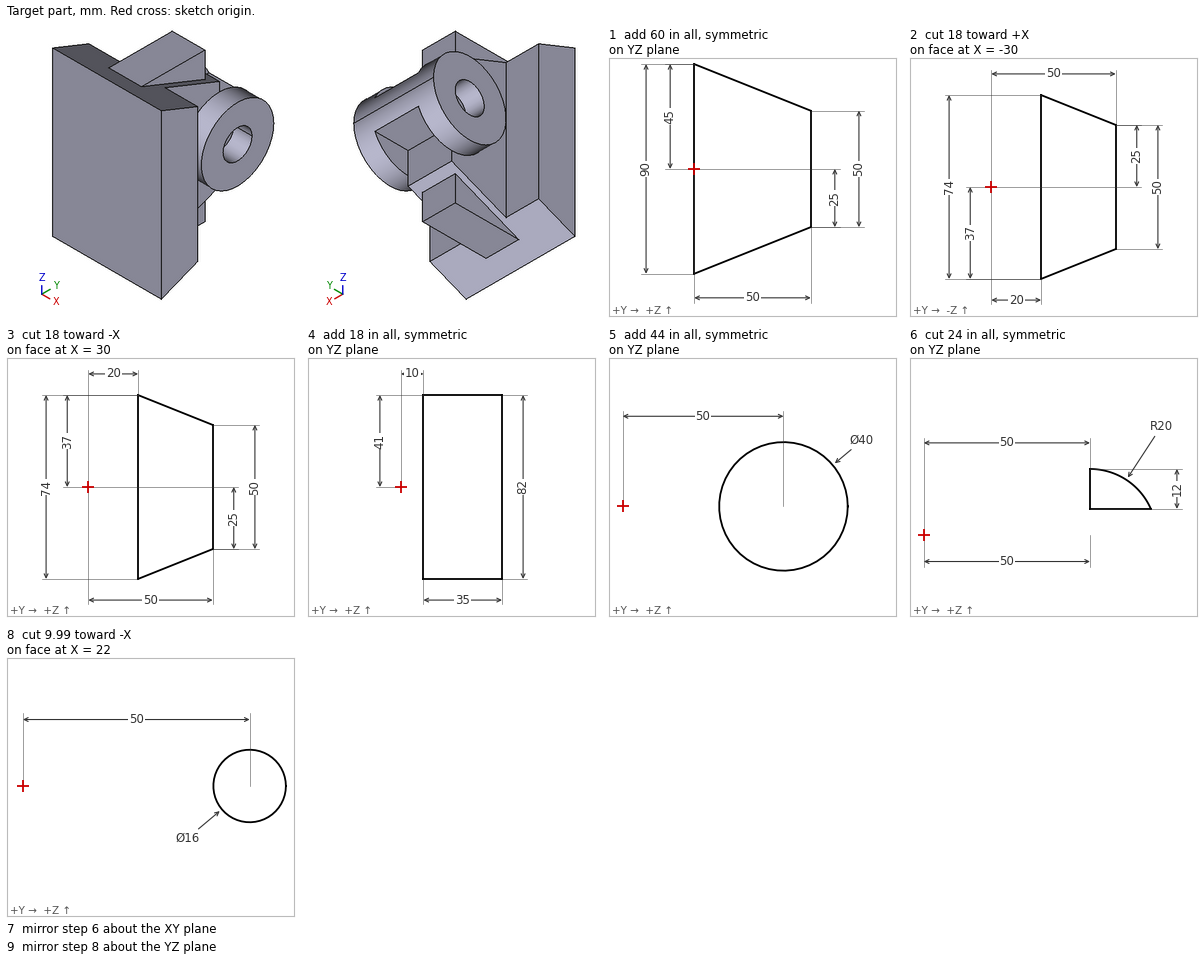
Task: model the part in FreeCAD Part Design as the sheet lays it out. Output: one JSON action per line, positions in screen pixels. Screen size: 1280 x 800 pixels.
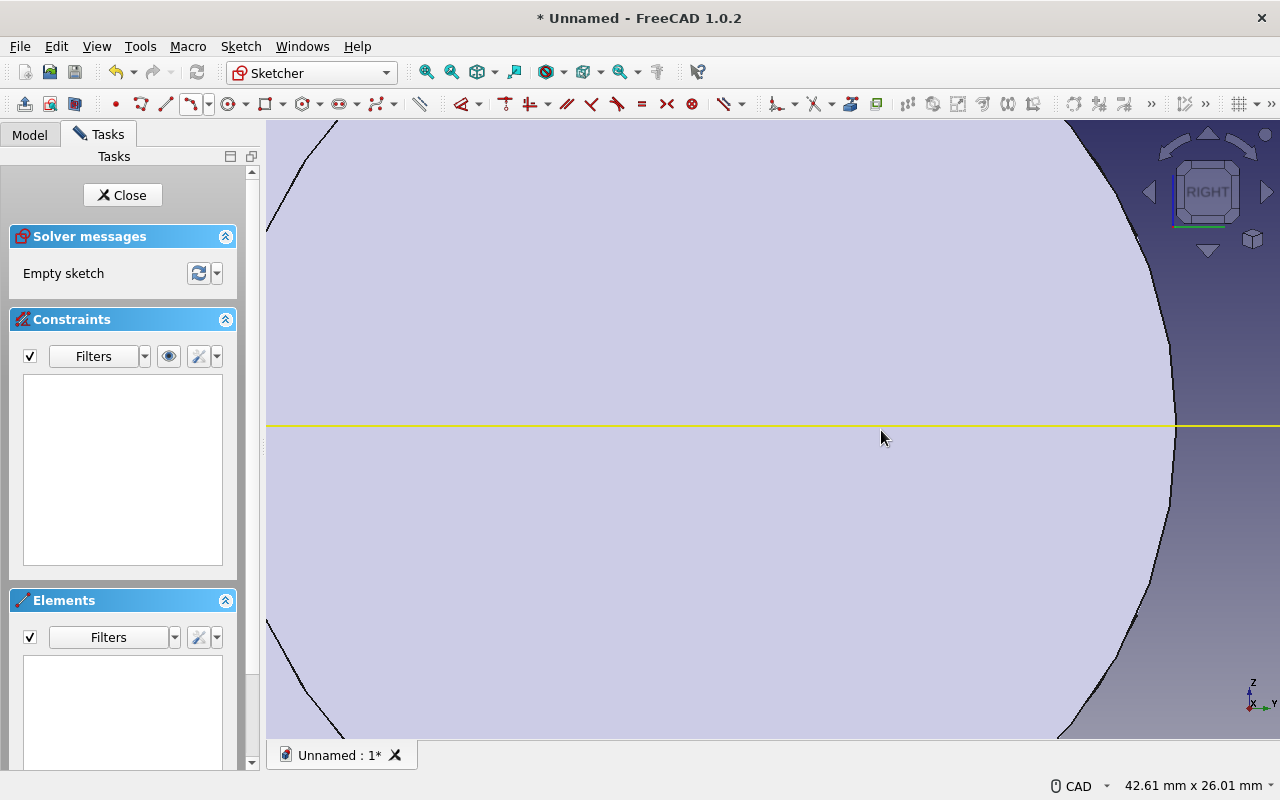
{"action": "left_click", "coordinate": [228, 104]}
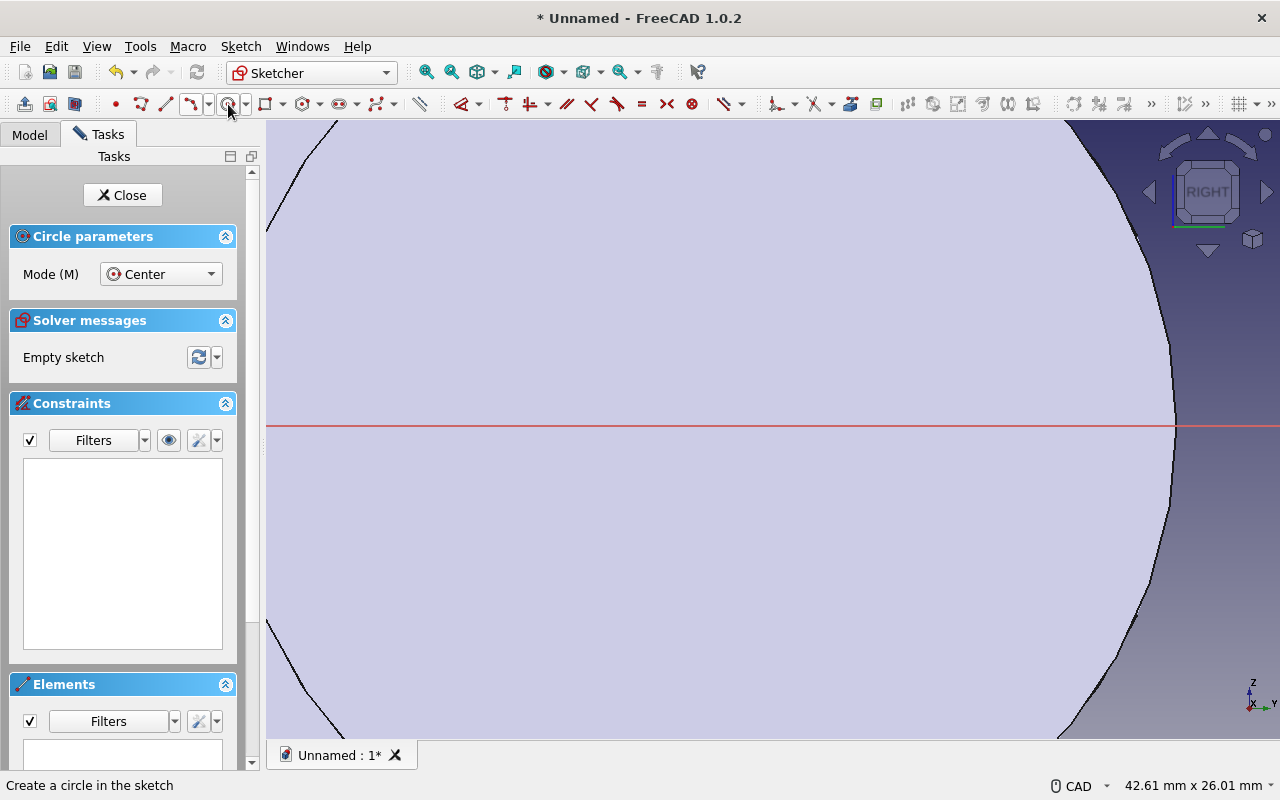
{"action": "left_click", "coordinate": [701, 426]}
{"action": "mouse_move", "coordinate": [835, 291]}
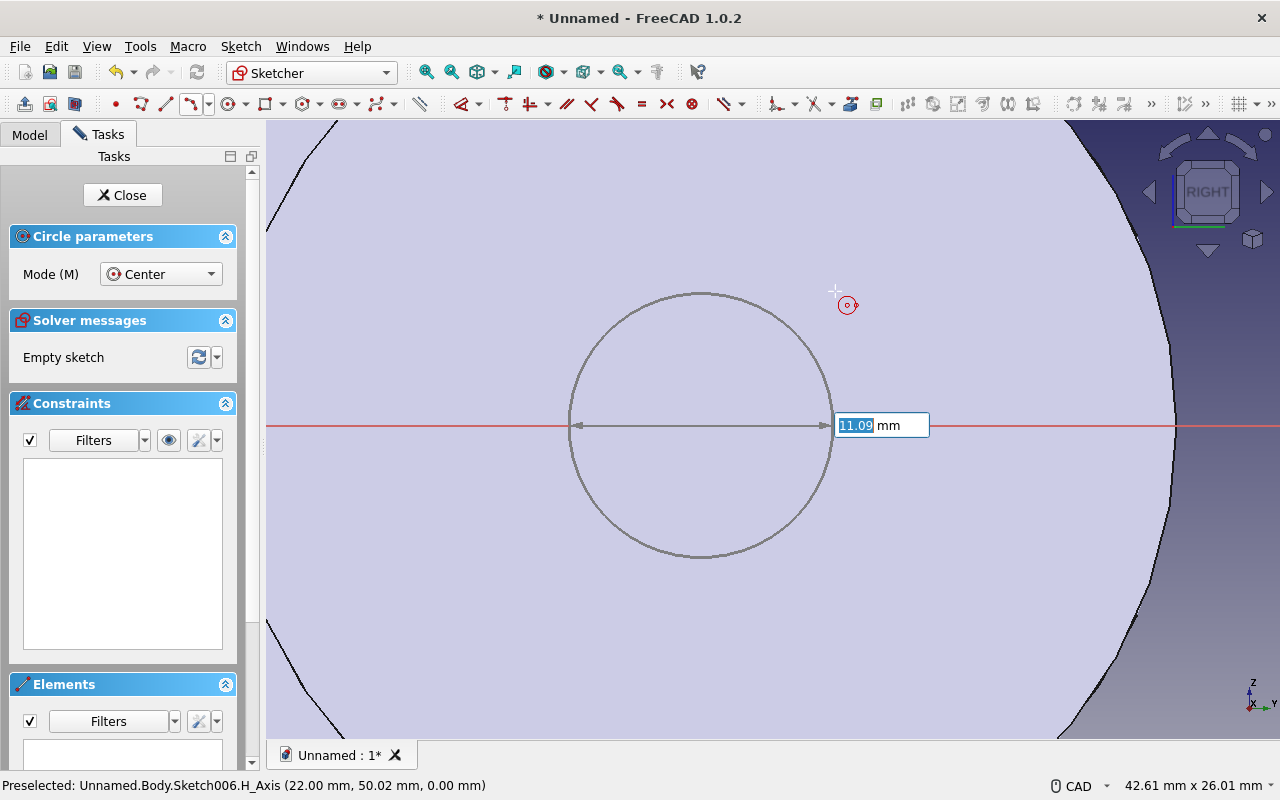
{"action": "type", "text": "16"}
{"action": "key", "text": "Return"}
{"action": "key", "text": "Escape"}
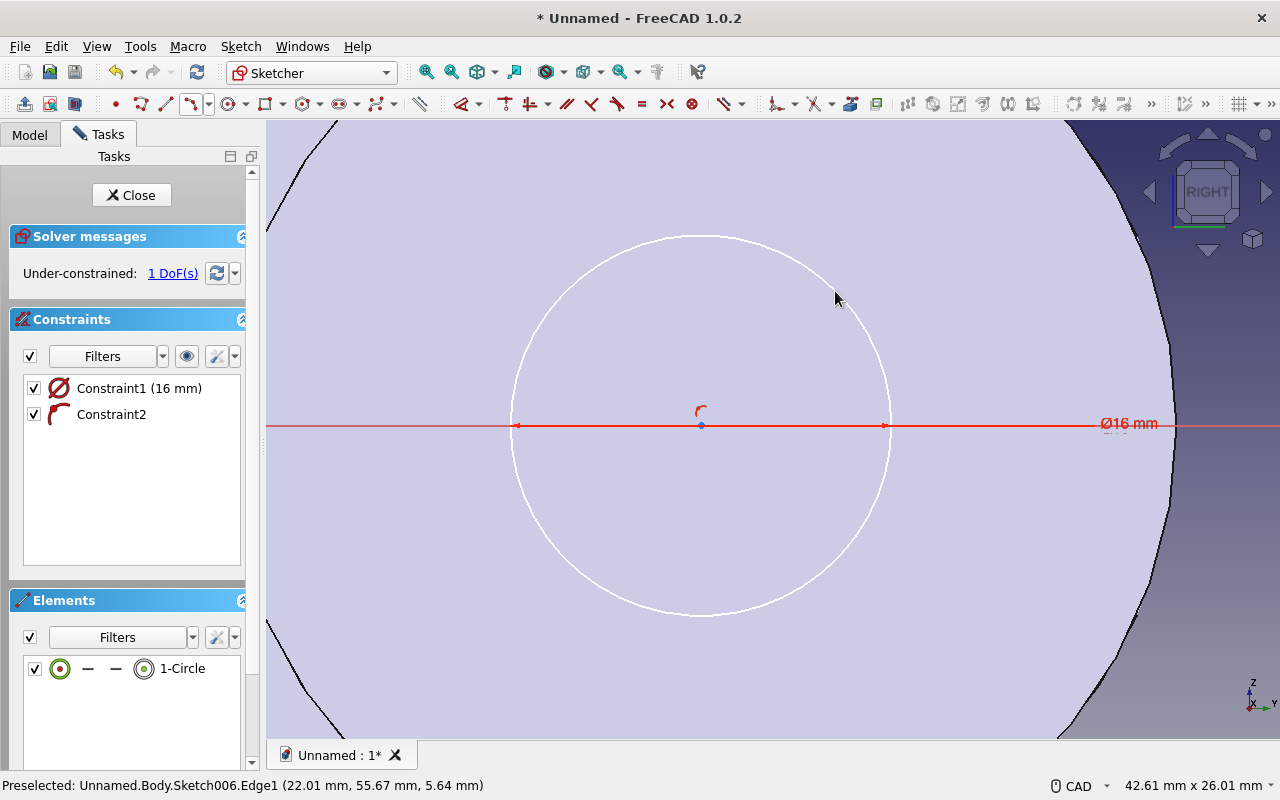
{"action": "left_click", "coordinate": [460, 104]}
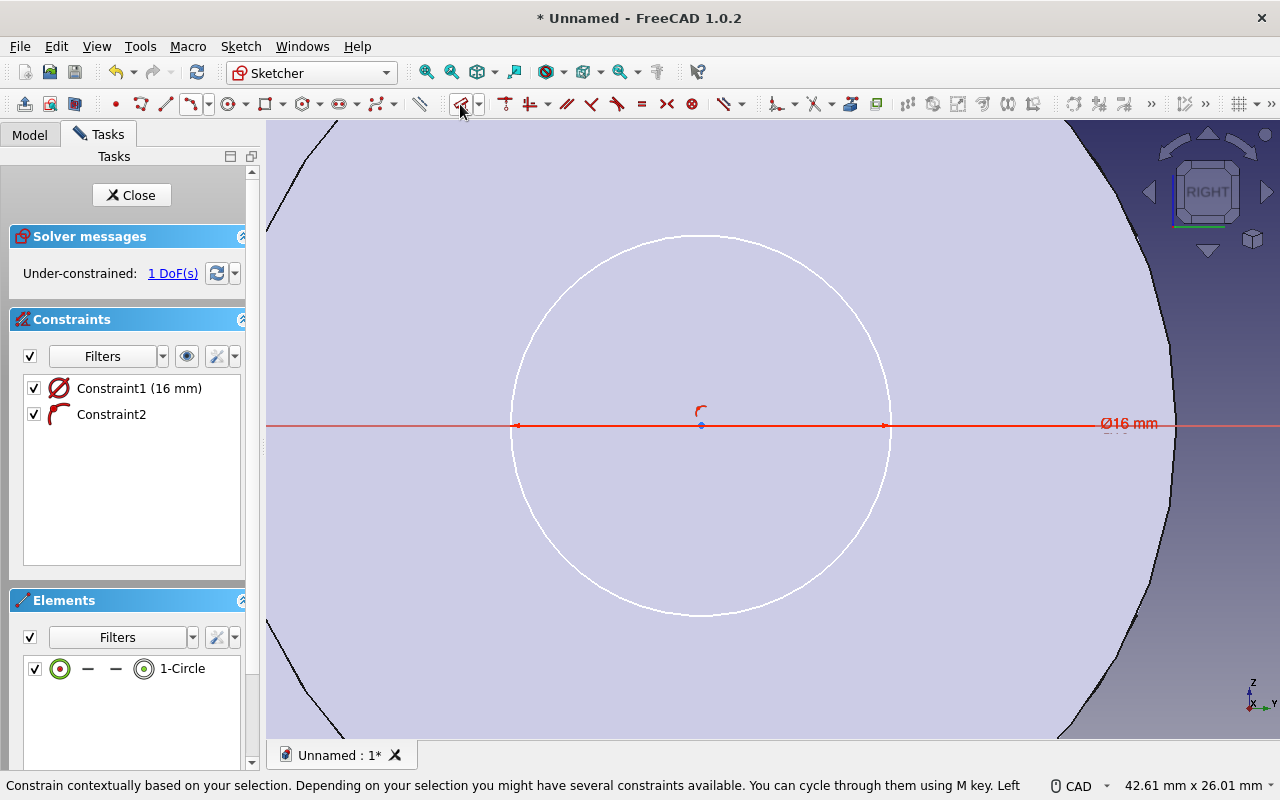
{"action": "left_click", "coordinate": [701, 426]}
{"action": "left_click", "coordinate": [498, 460]}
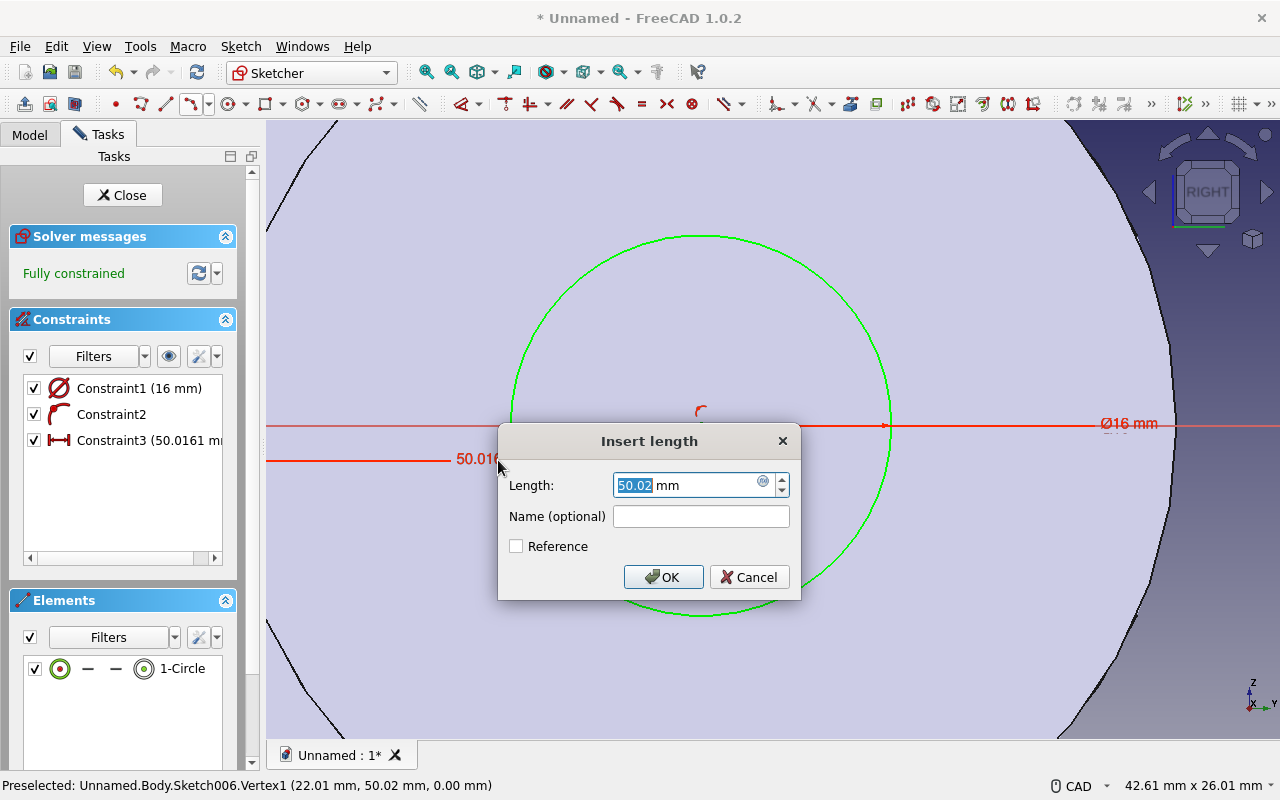
{"action": "type", "text": "50"}
{"action": "key", "text": "Return"}
{"action": "key", "text": "Escape"}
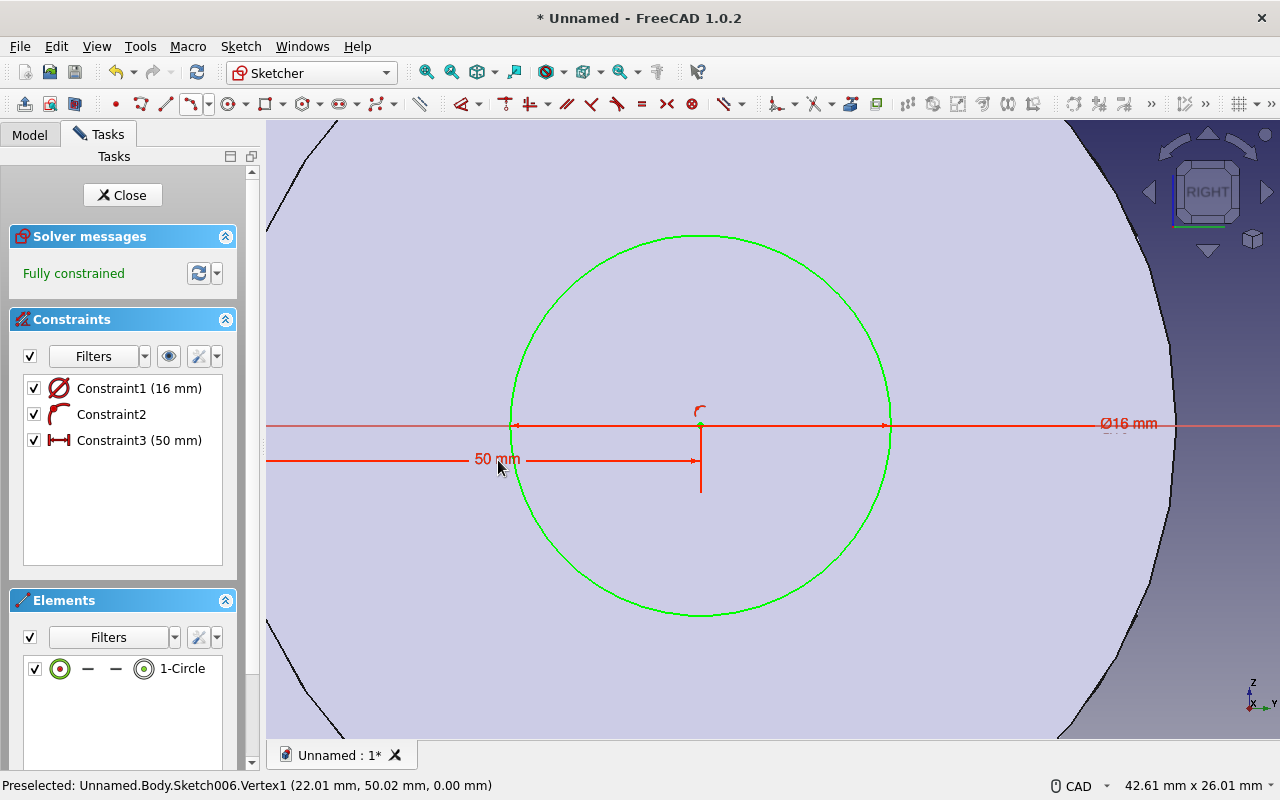
{"action": "left_click", "coordinate": [123, 195]}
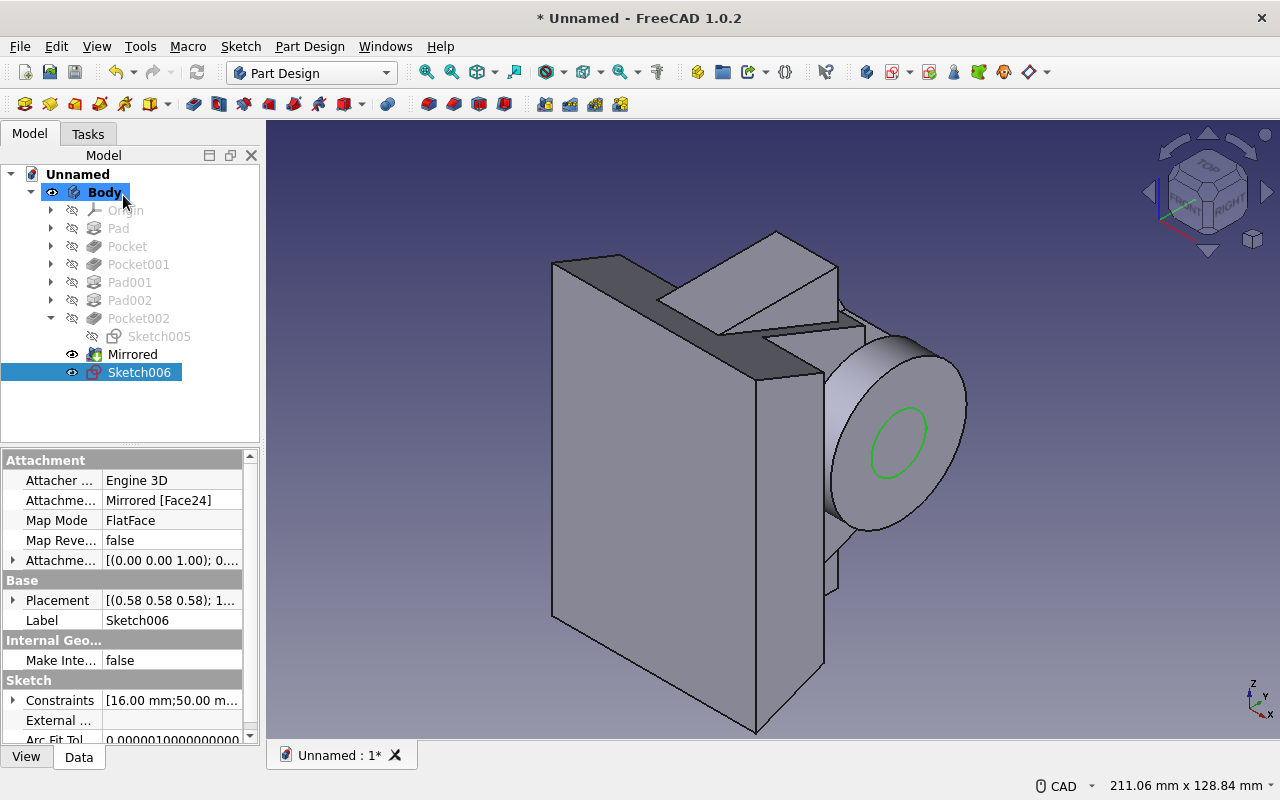
{"action": "left_click", "coordinate": [194, 104]}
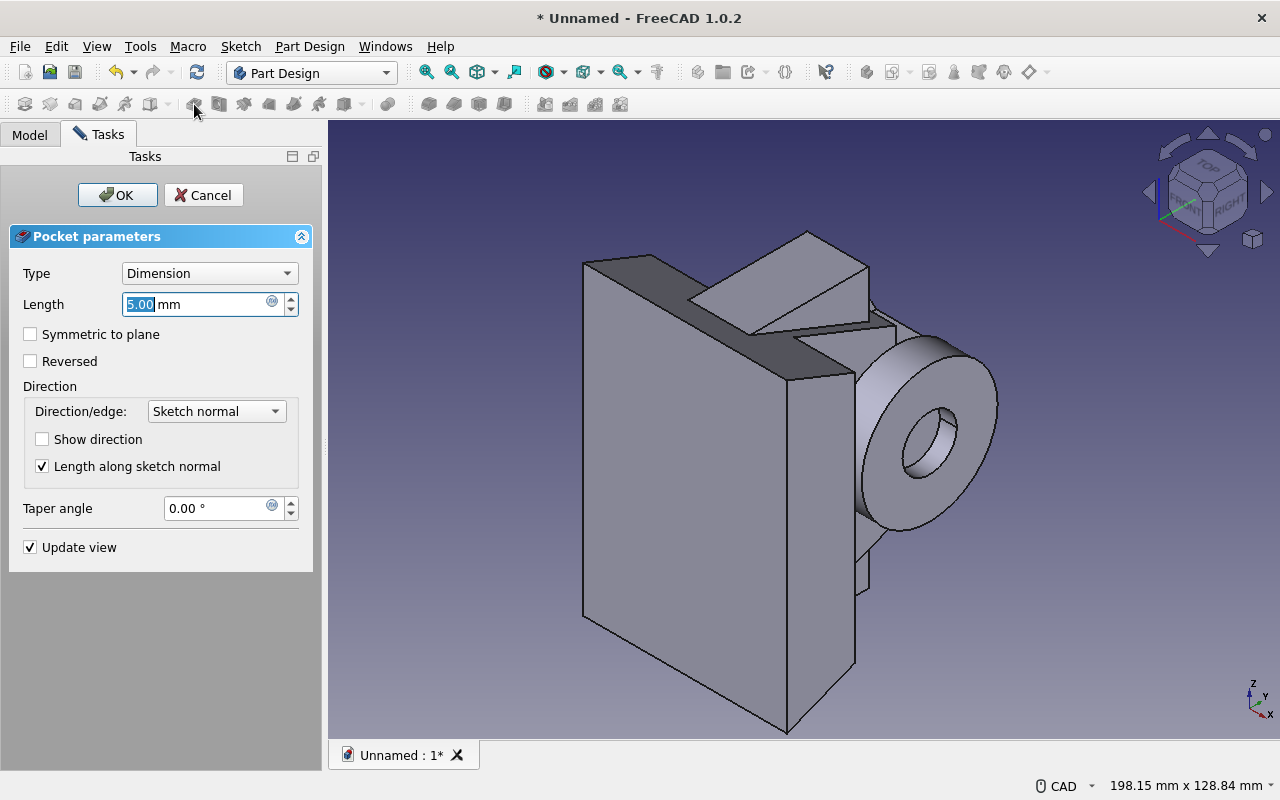
{"action": "type", "text": "9.99"}
{"action": "key", "text": "Tab"}